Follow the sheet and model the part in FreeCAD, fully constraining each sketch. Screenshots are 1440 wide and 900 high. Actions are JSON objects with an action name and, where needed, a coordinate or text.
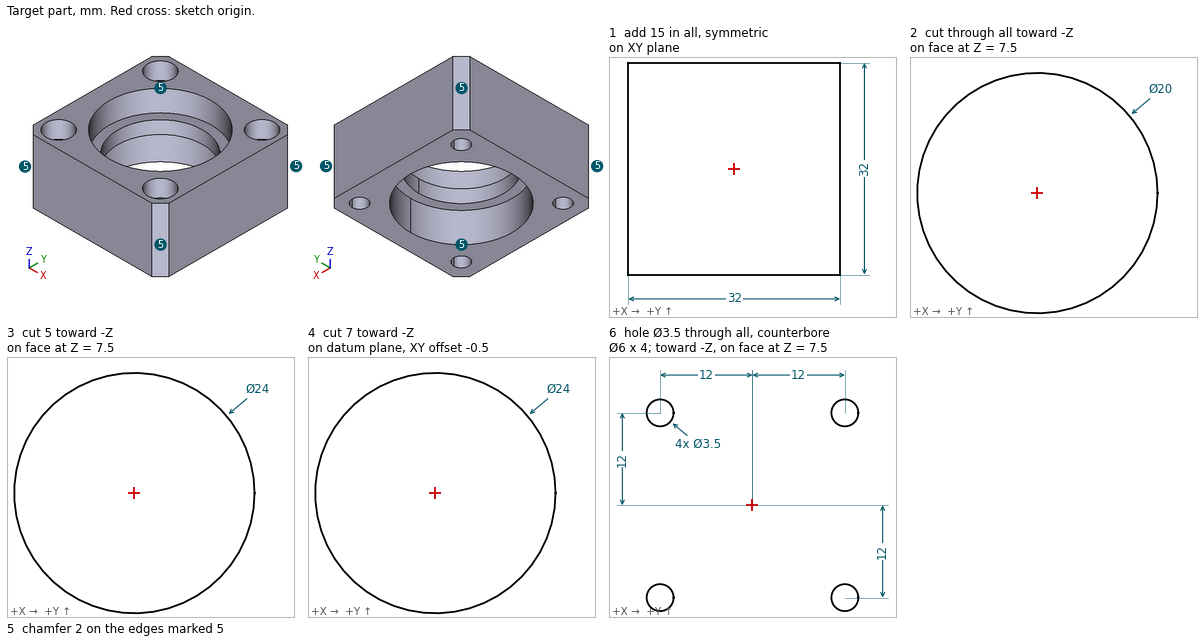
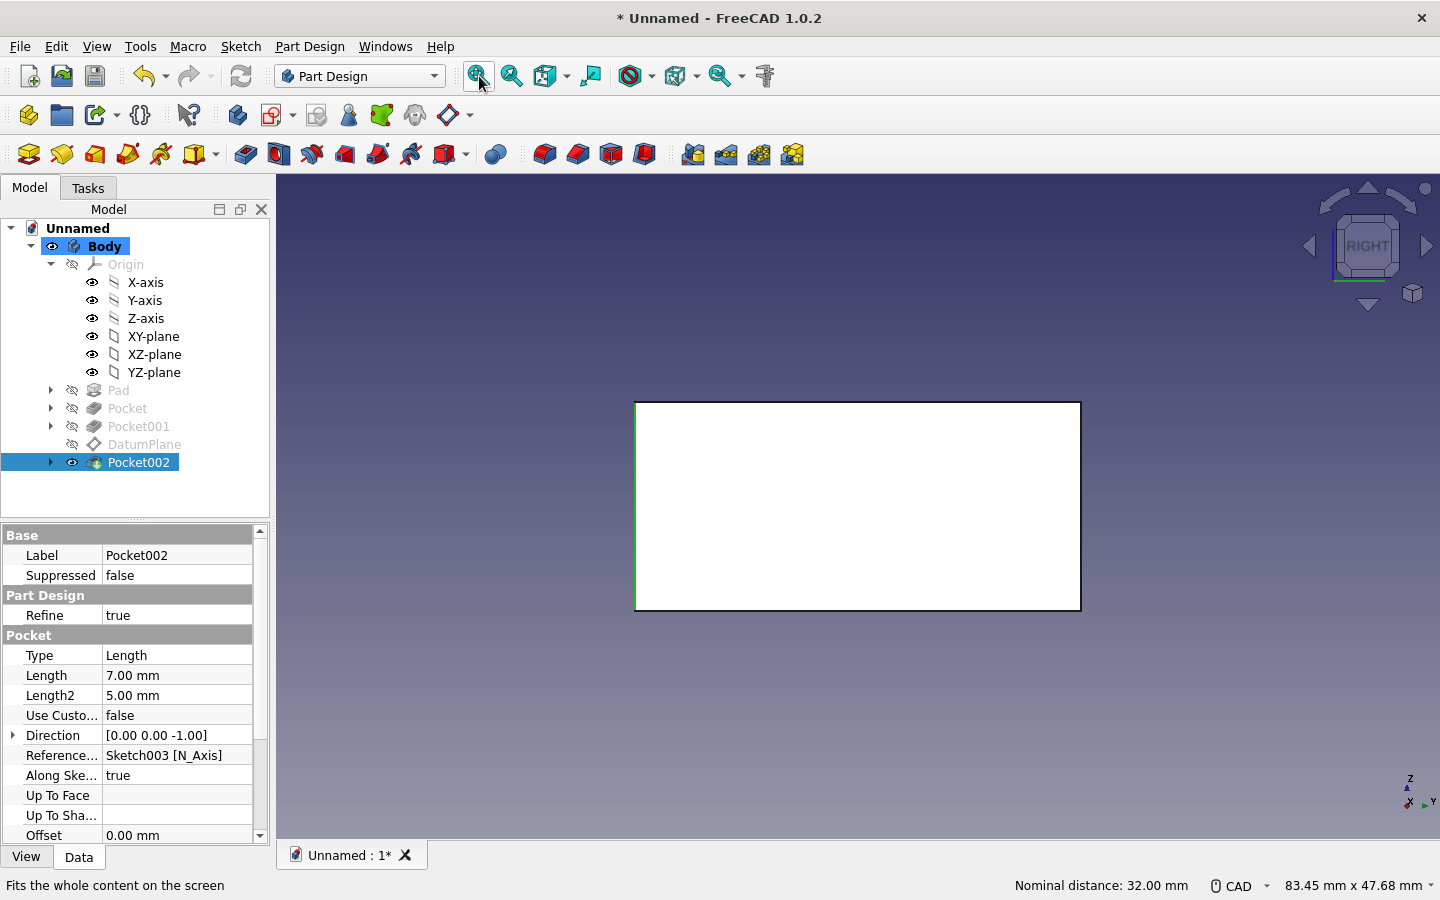
{"action": "left_click", "coordinate": [1081, 505], "text": "ctrl"}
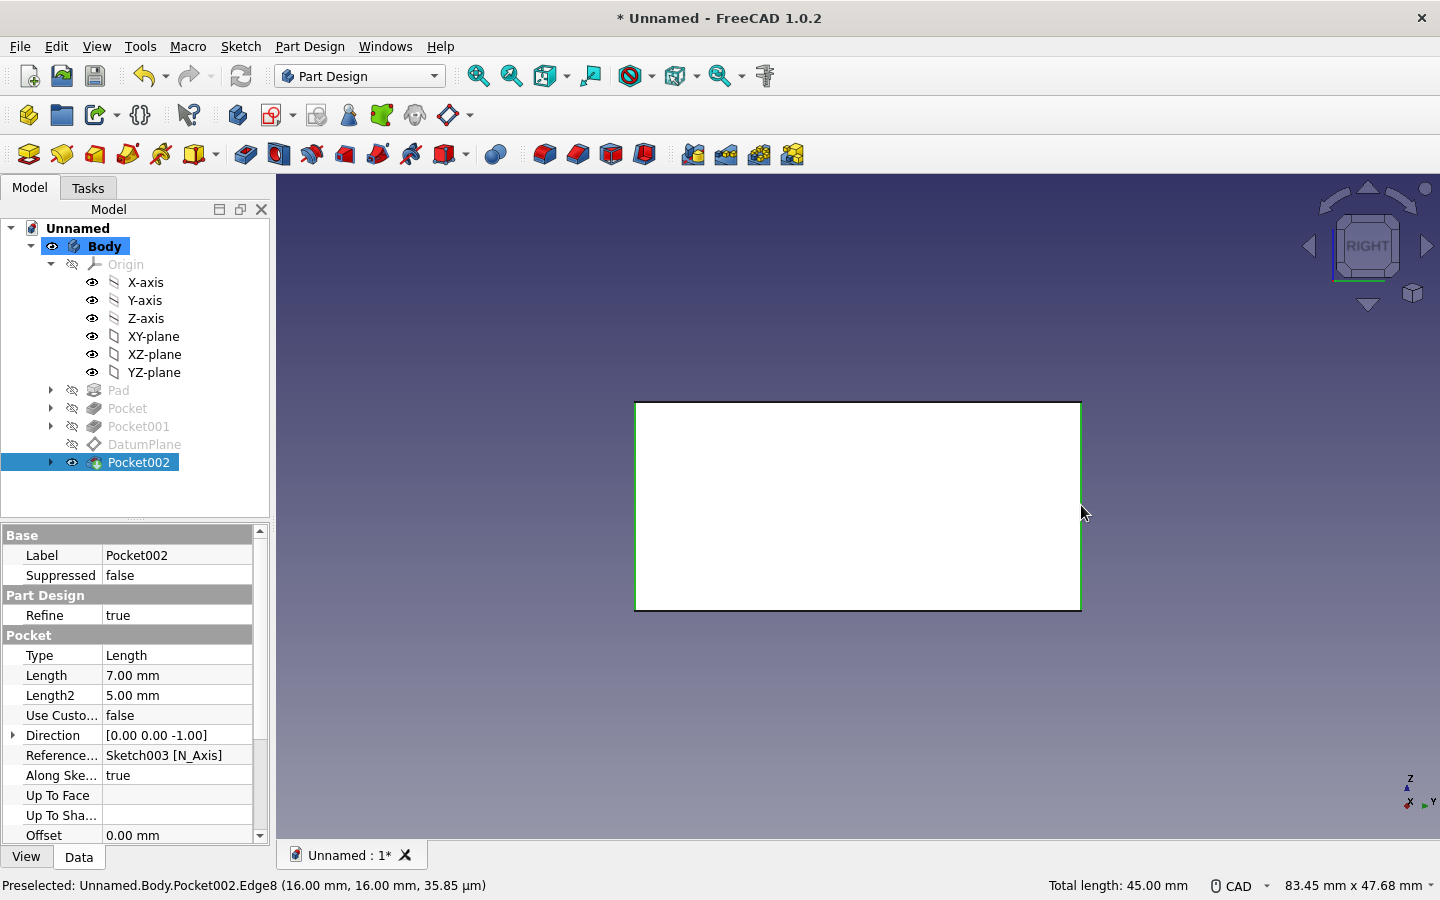
{"action": "key", "text": "5"}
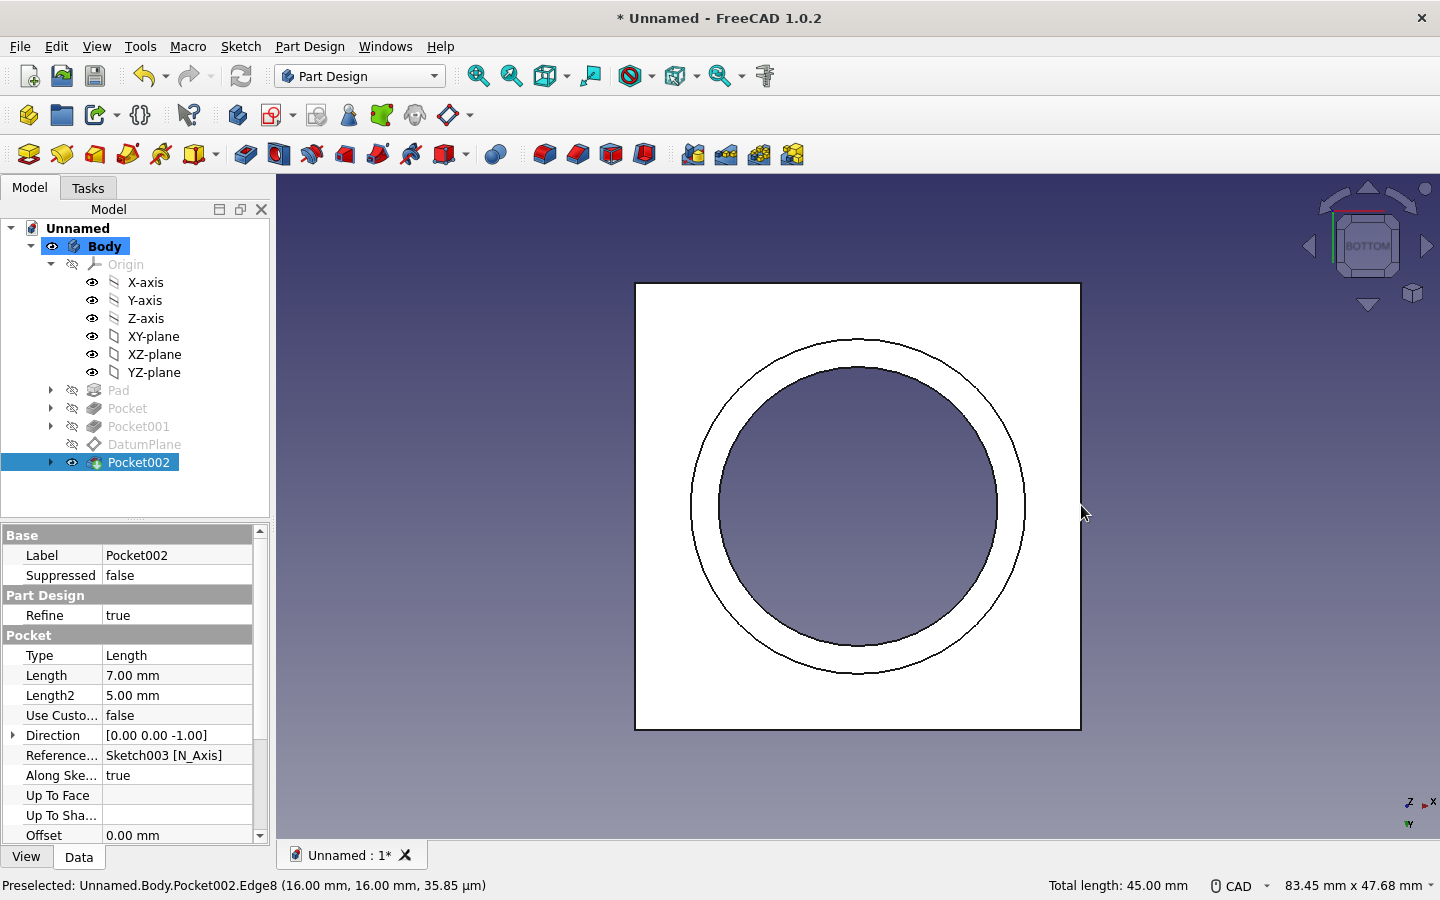
{"action": "key", "text": "4"}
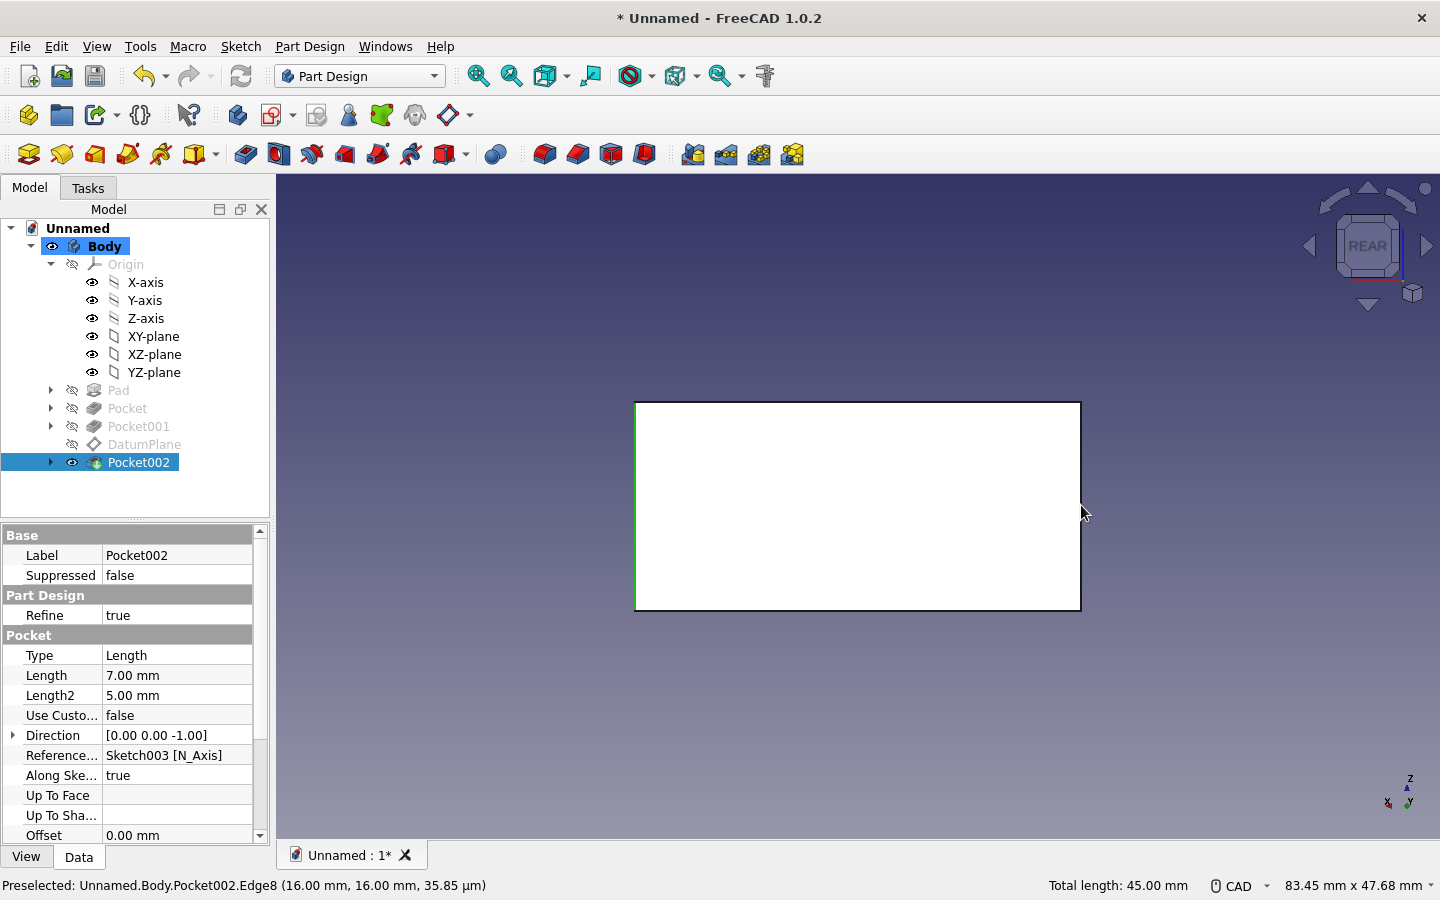
{"action": "key", "text": "v f"}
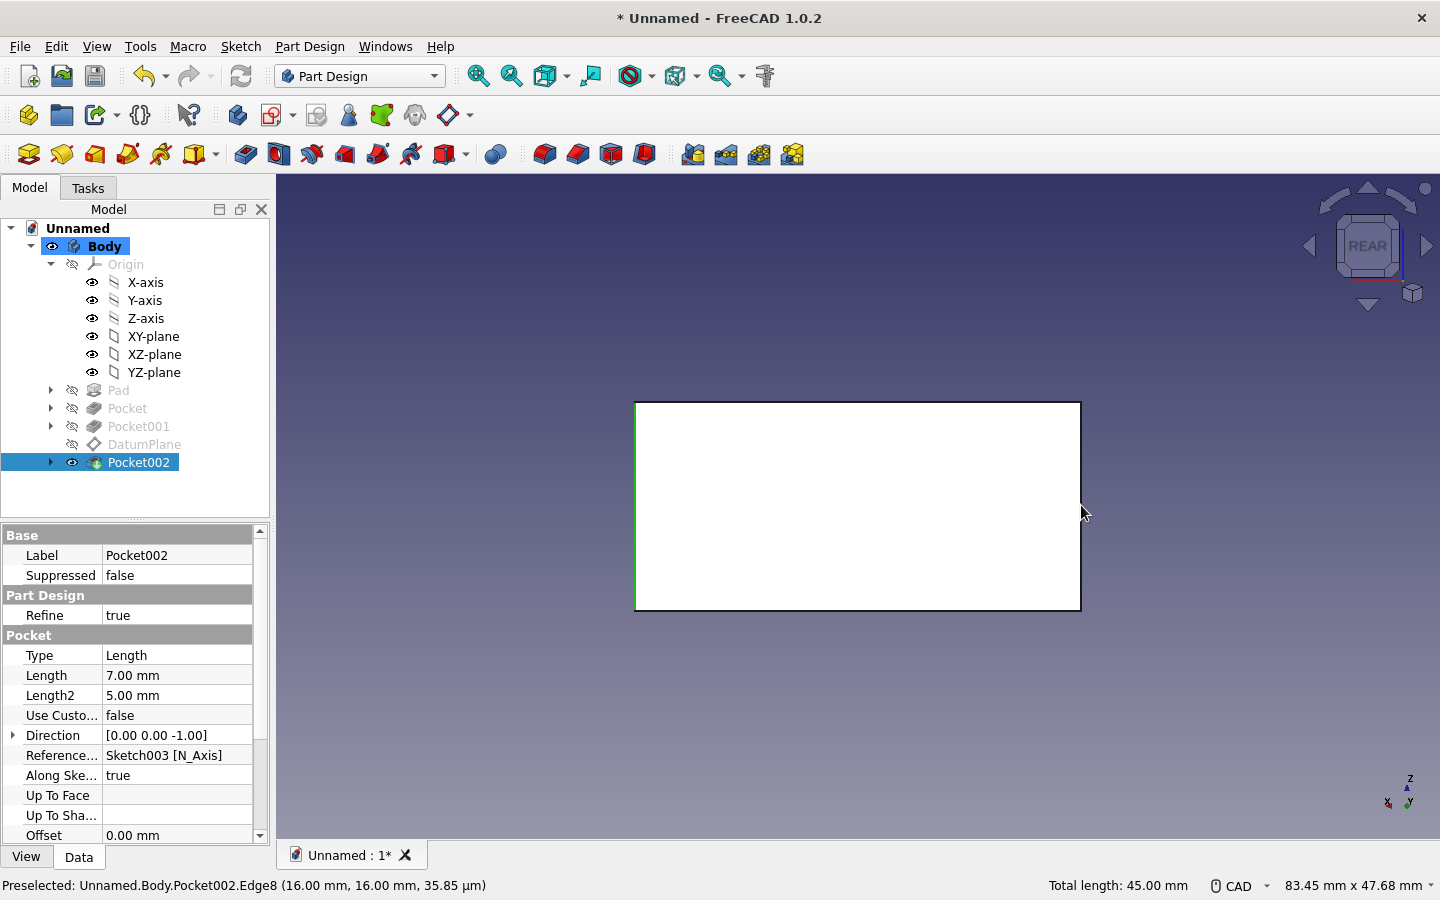
{"action": "left_click", "coordinate": [1081, 506], "text": "ctrl"}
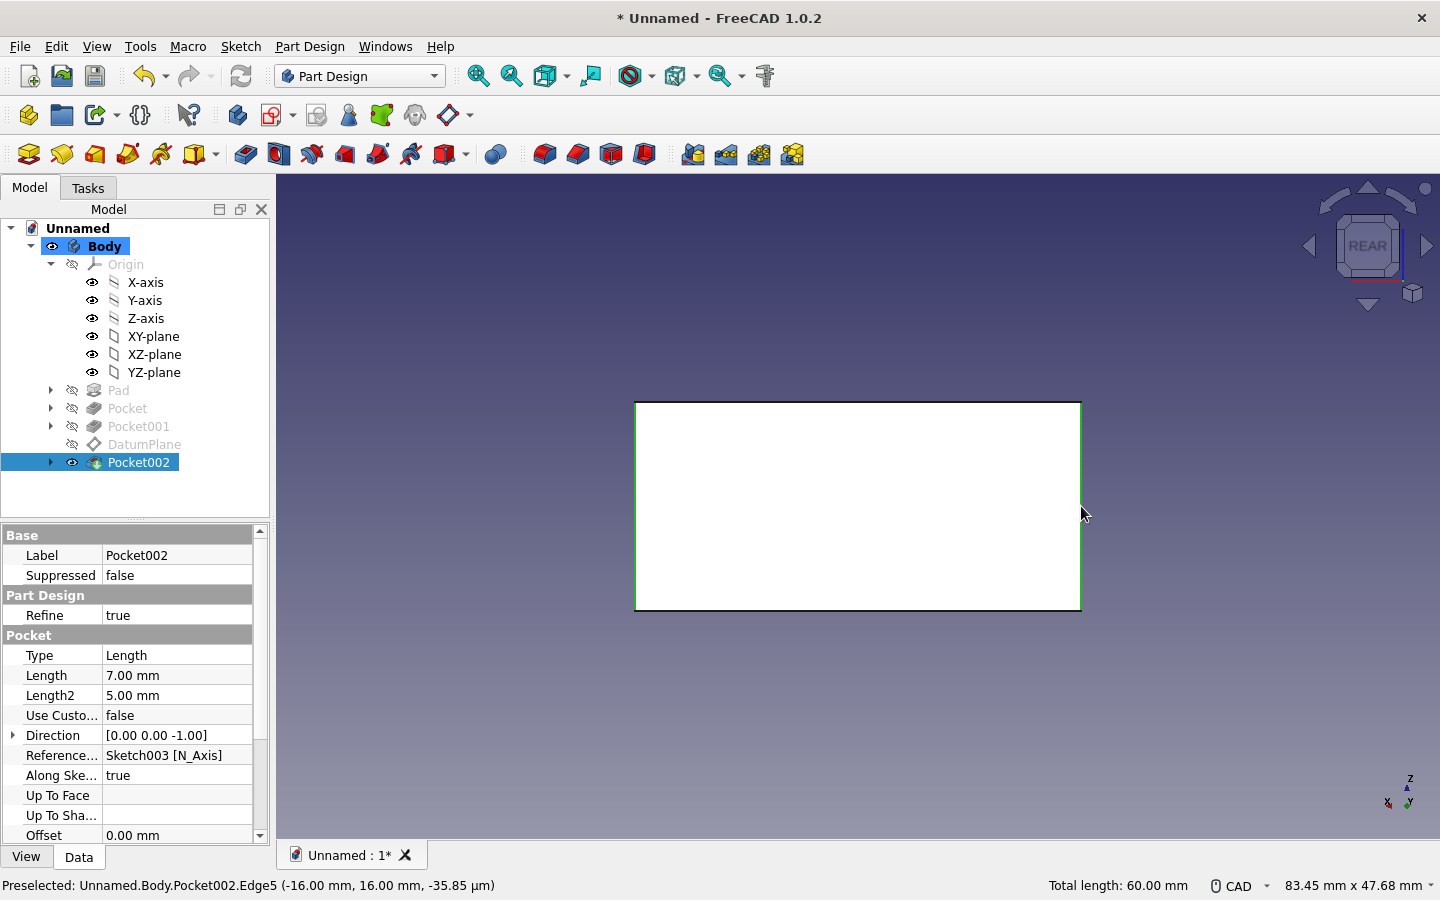
{"action": "left_click", "coordinate": [578, 154]}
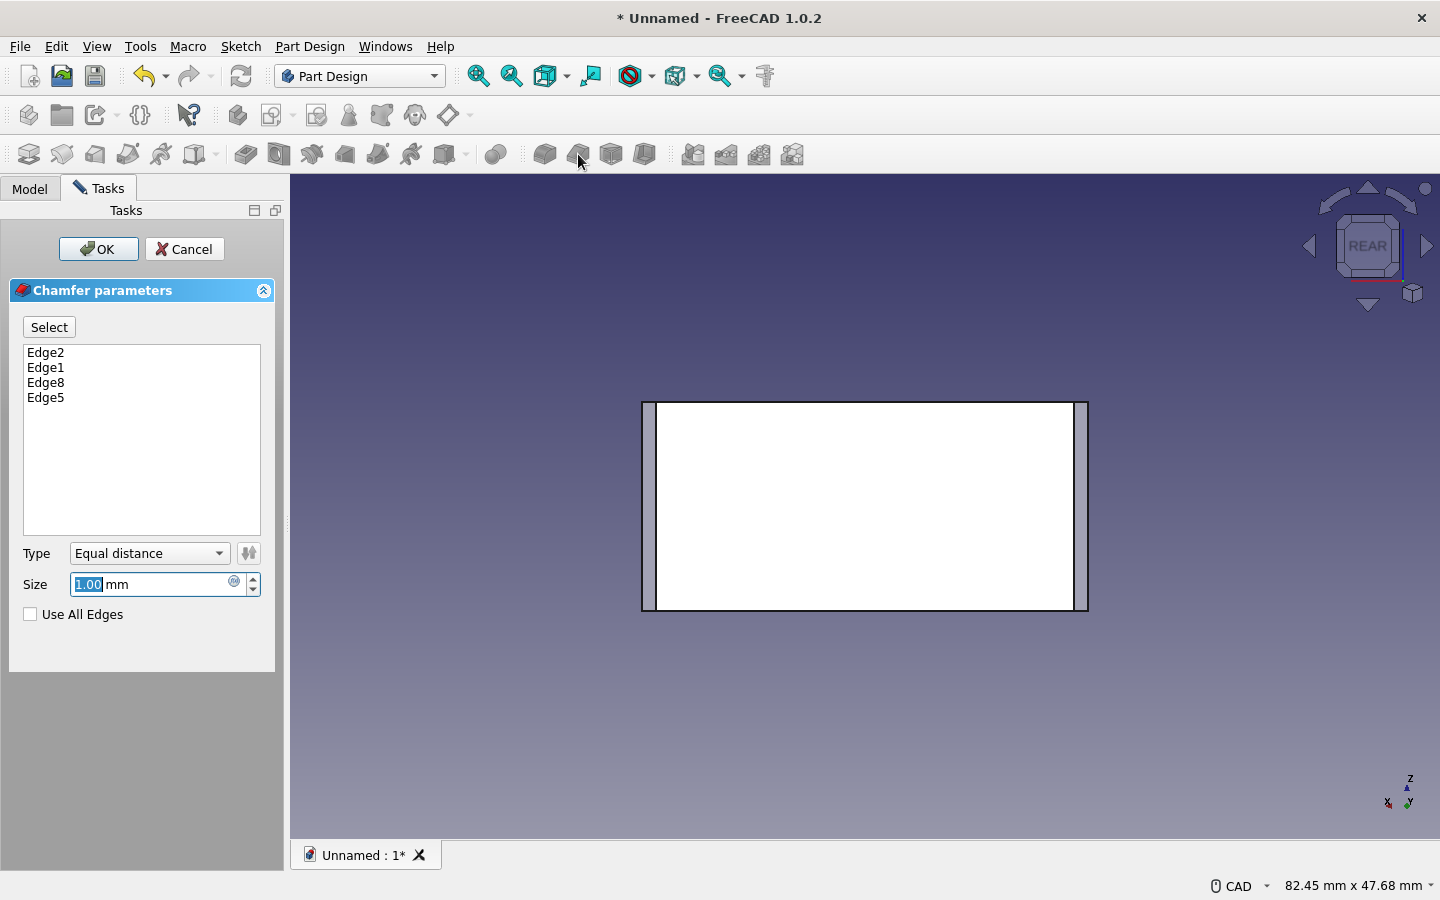
{"action": "type", "text": "2"}
{"action": "key", "text": "Tab"}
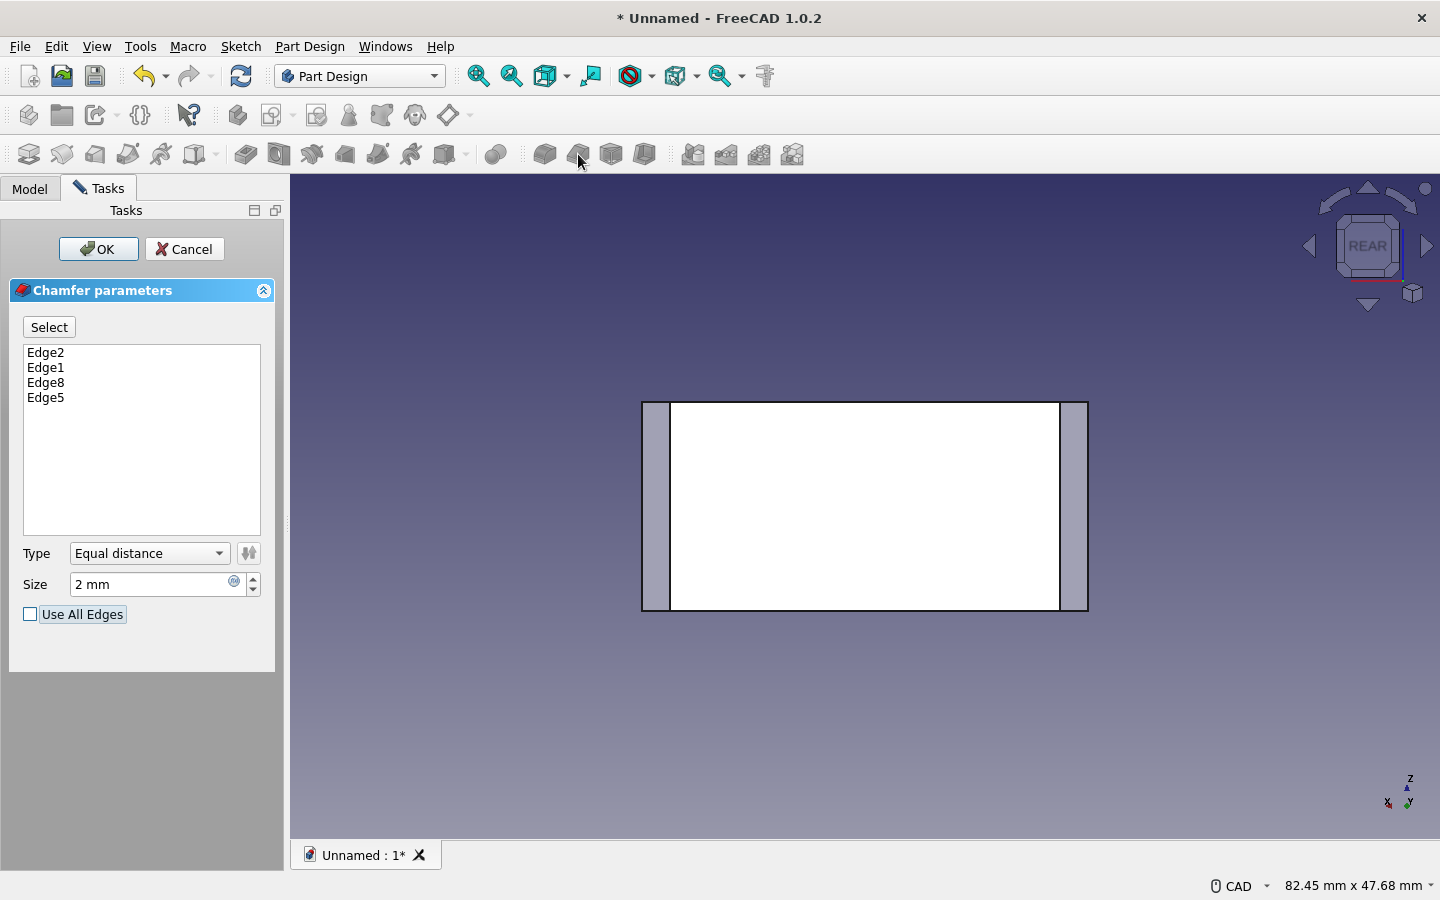
{"action": "left_click", "coordinate": [99, 249]}